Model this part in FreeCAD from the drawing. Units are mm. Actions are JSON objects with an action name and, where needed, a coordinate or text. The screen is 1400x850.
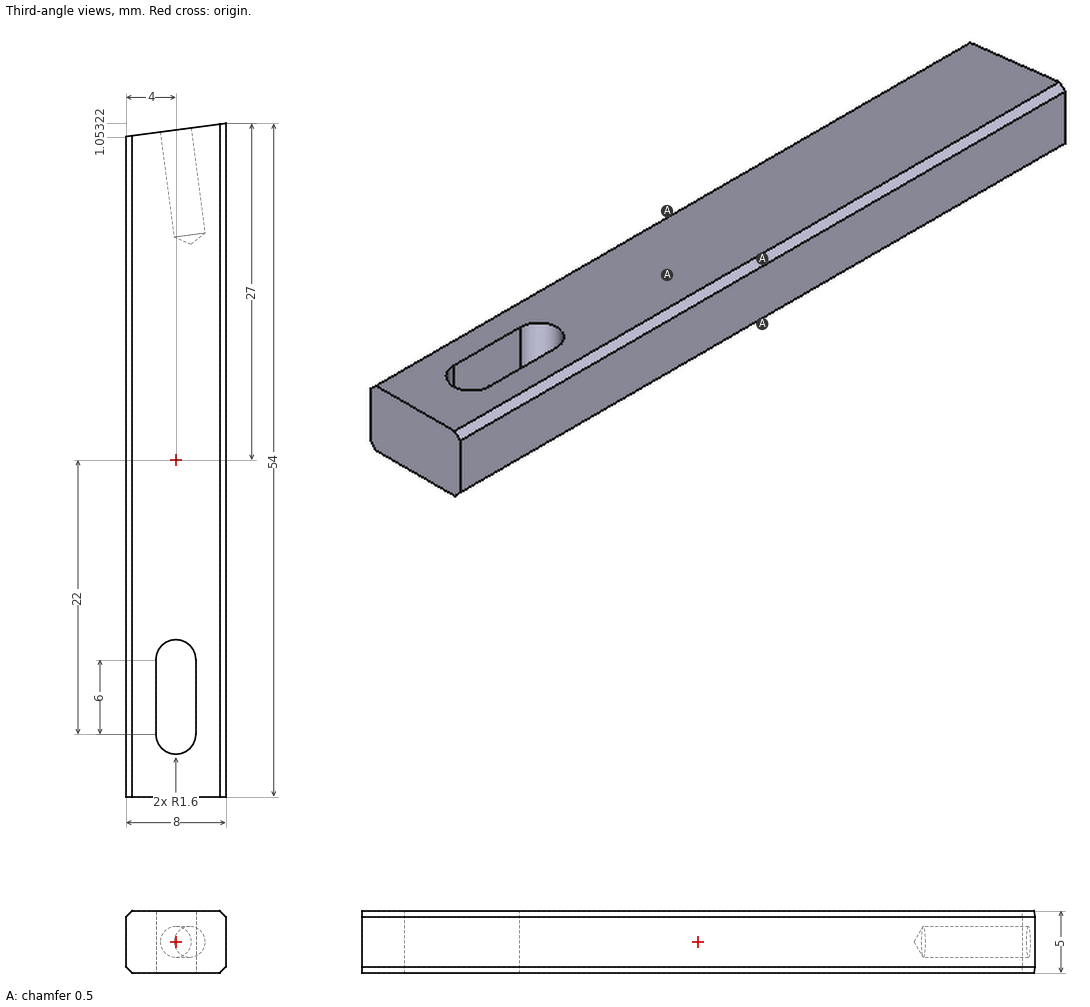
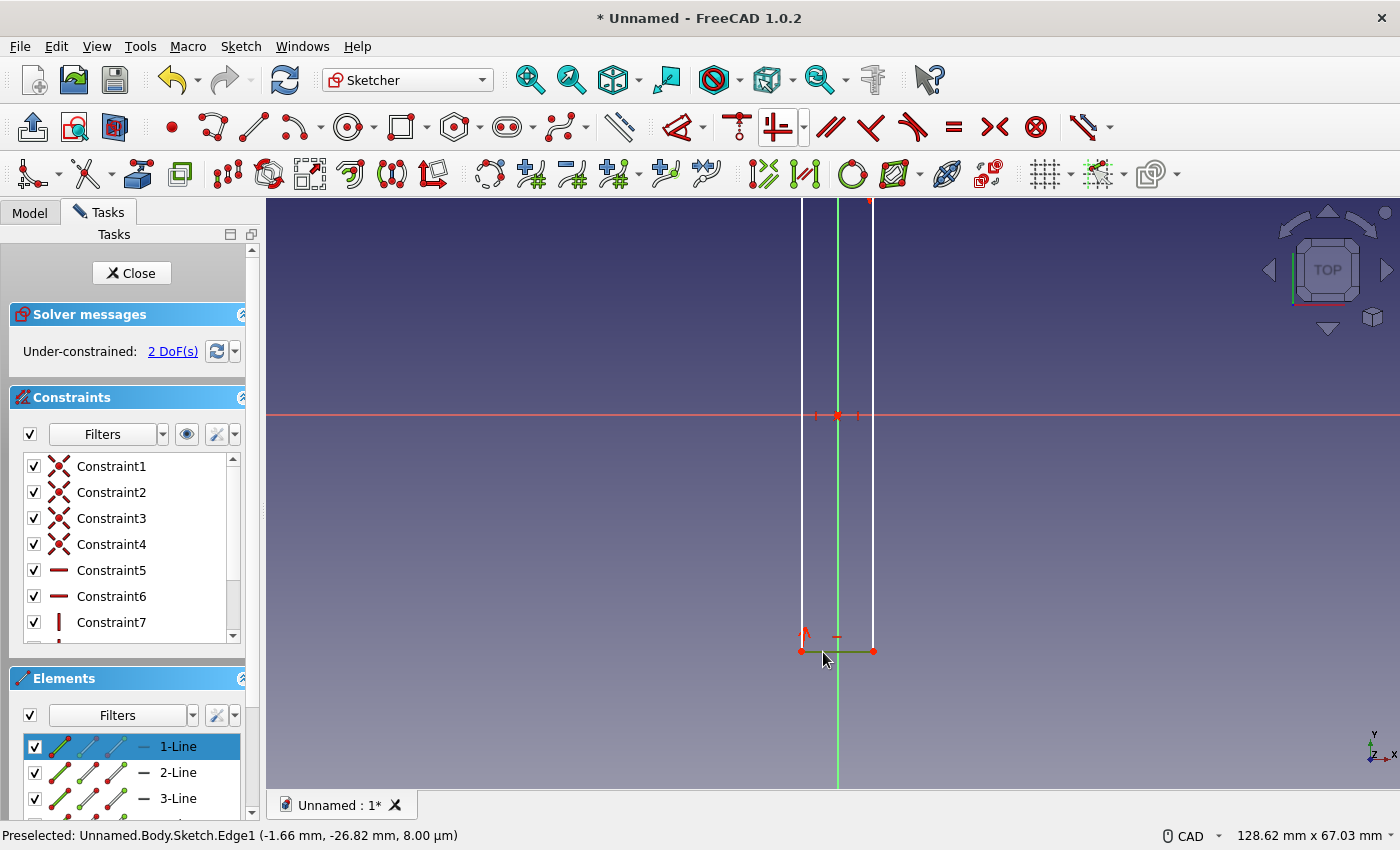
{"action": "key", "text": "l"}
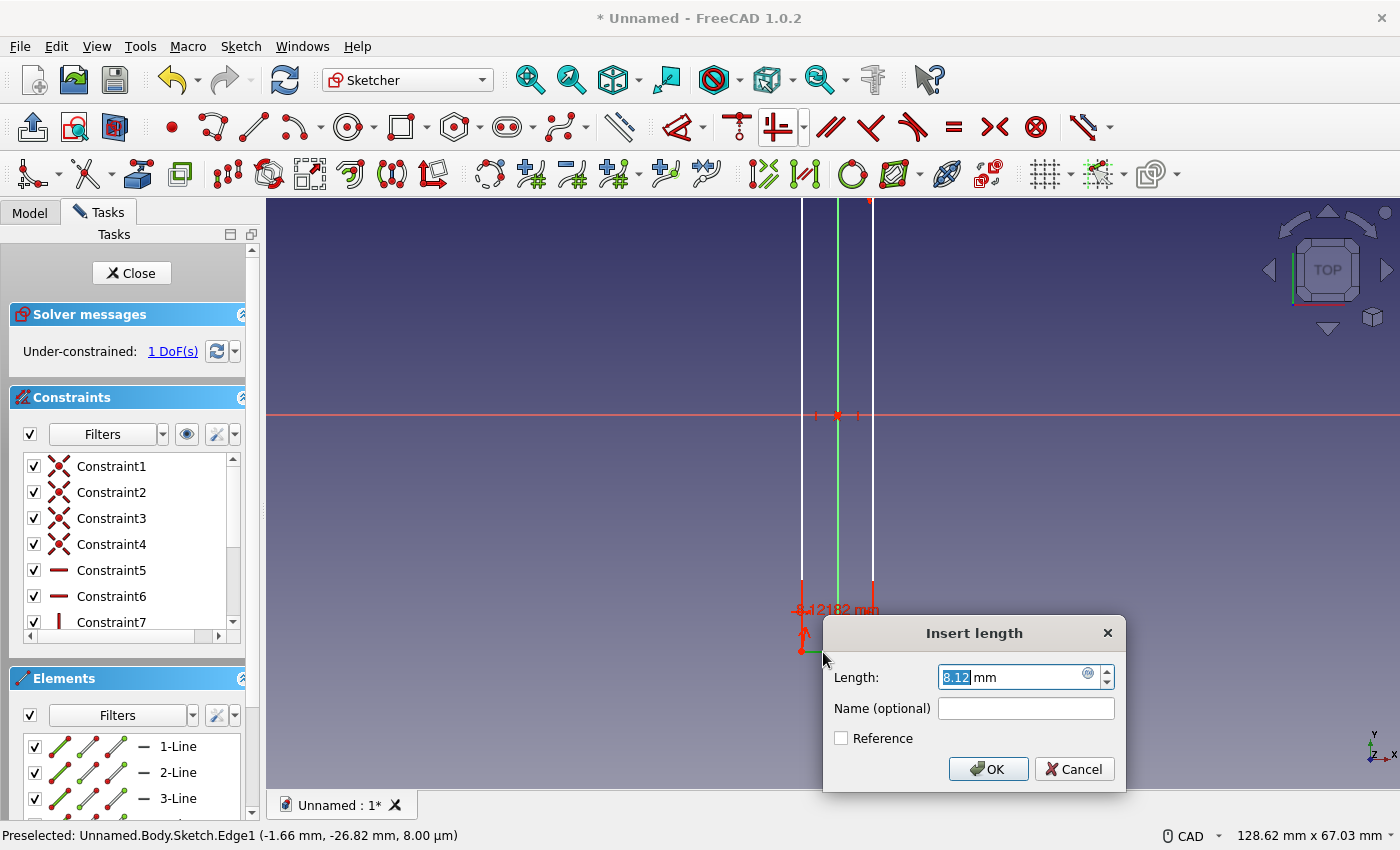
{"action": "type", "text": "8"}
{"action": "key", "text": "Return"}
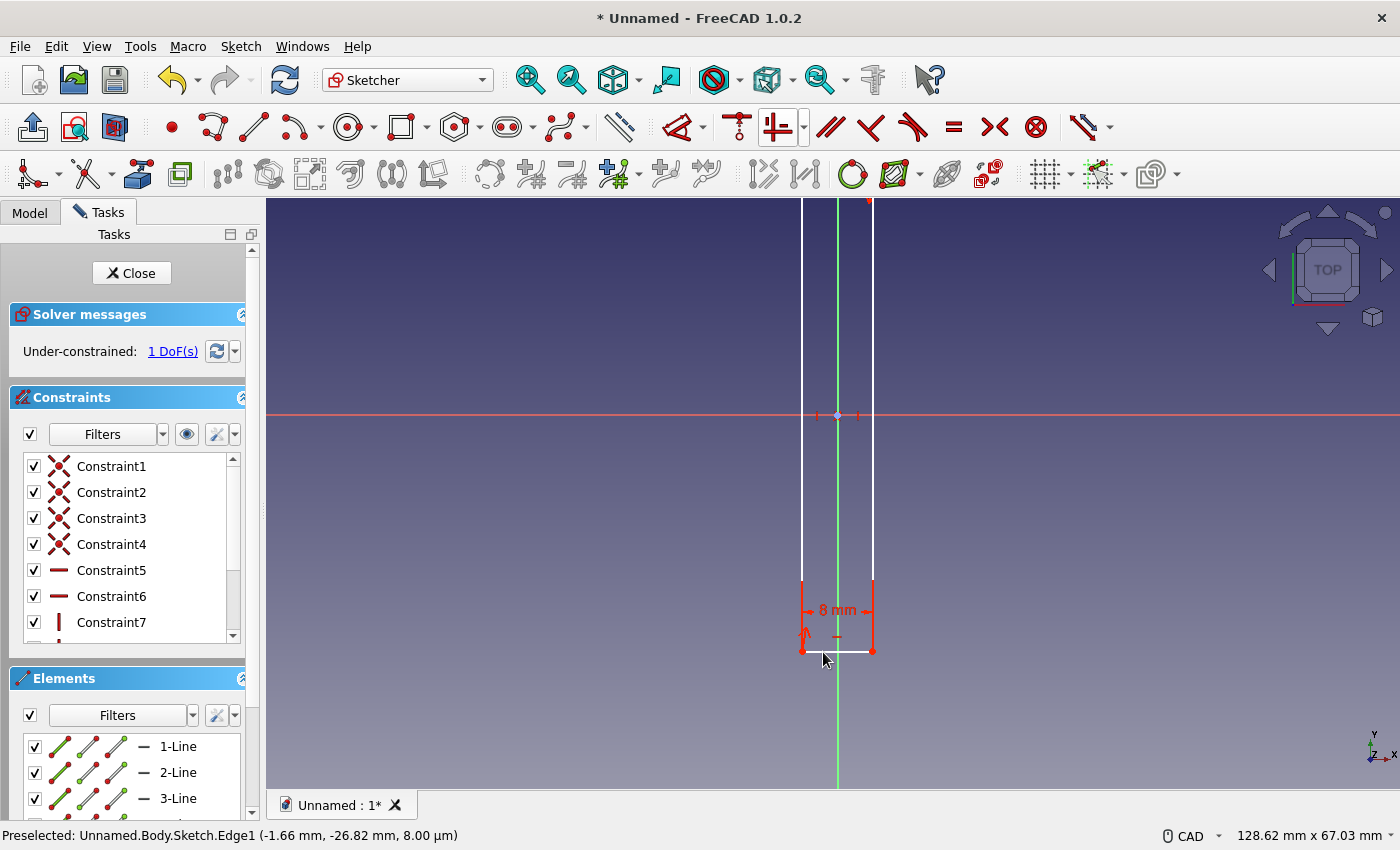
{"action": "left_click", "coordinate": [873, 510]}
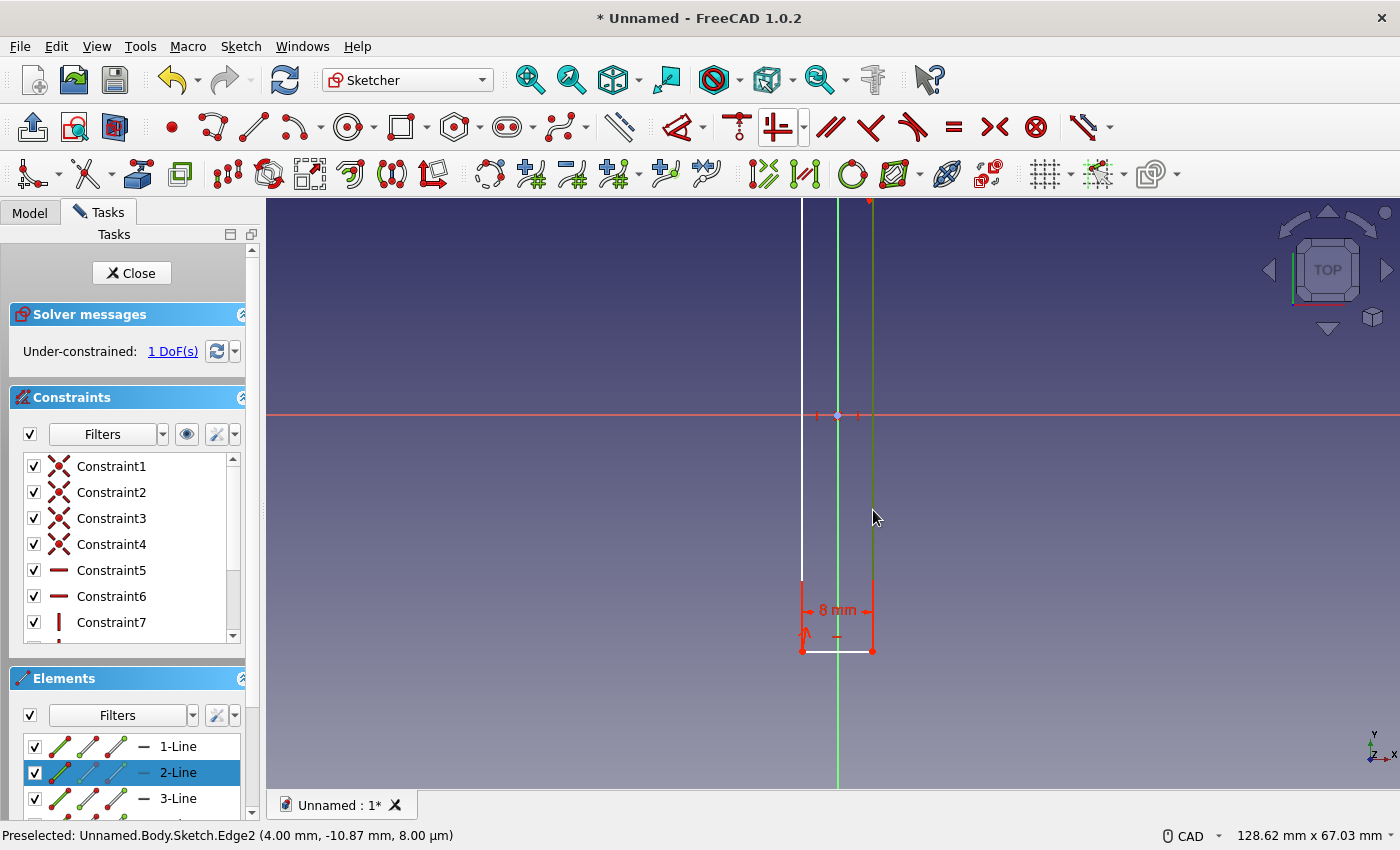
{"action": "key", "text": "i"}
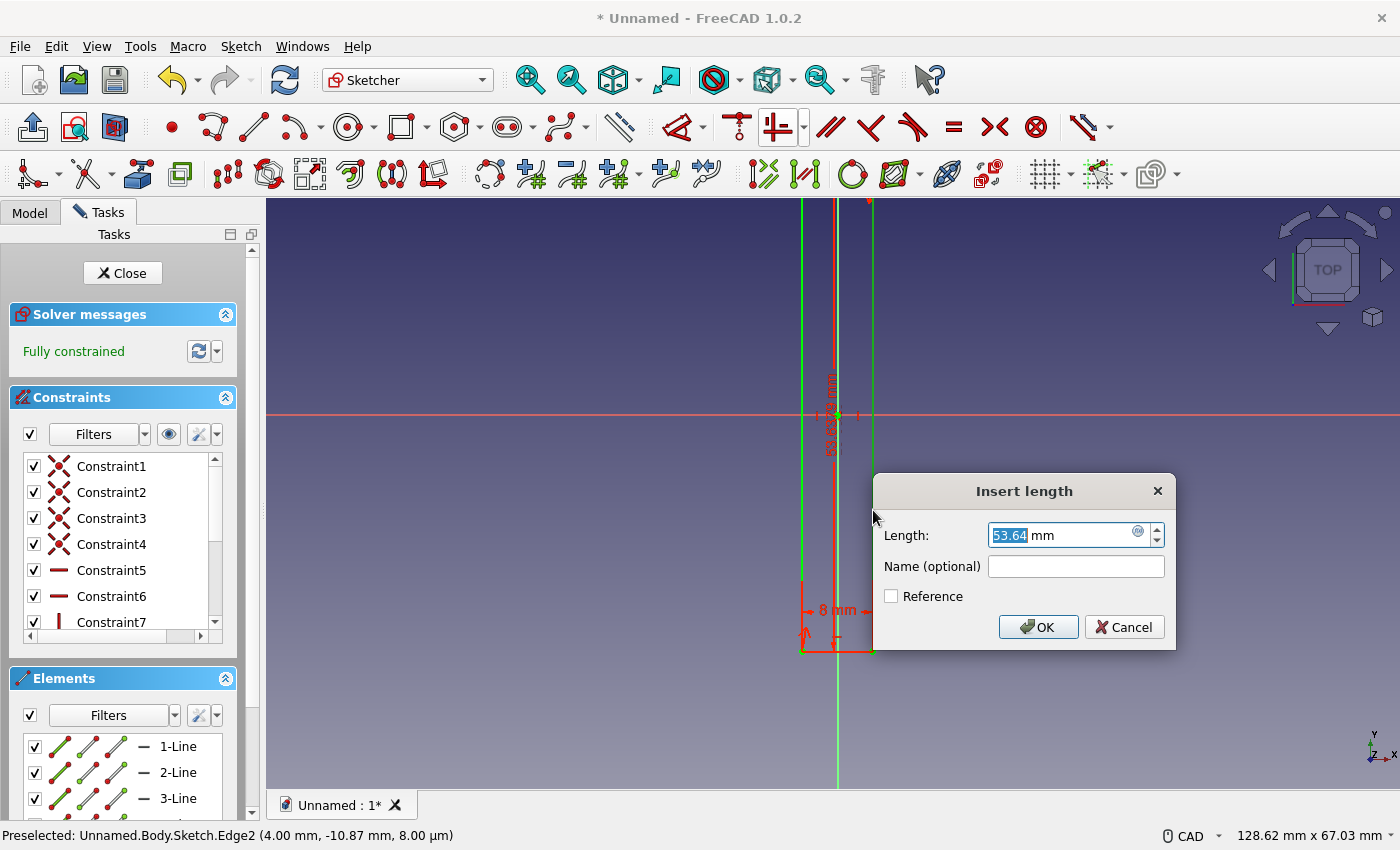
{"action": "type", "text": "54"}
{"action": "key", "text": "Return"}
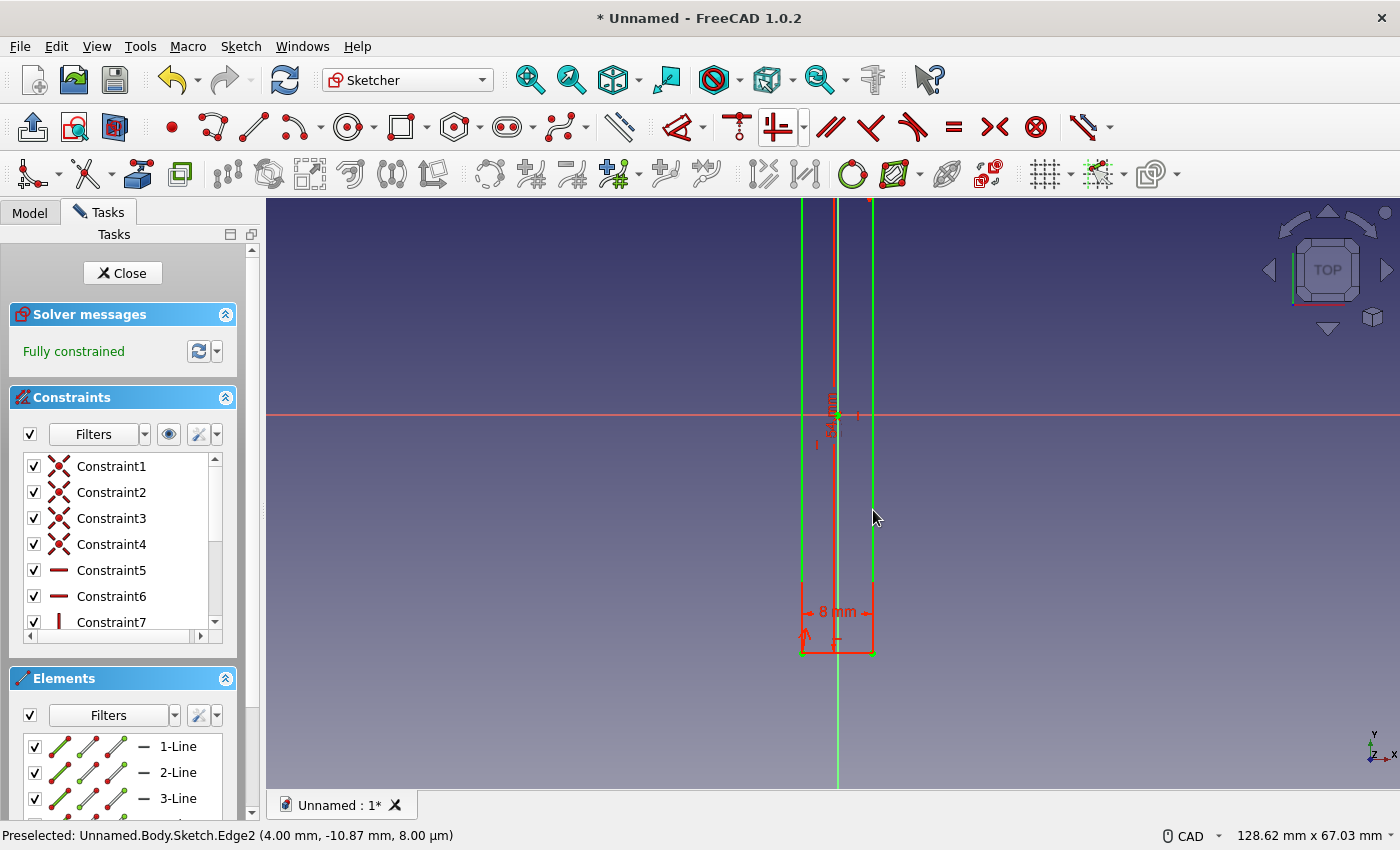
{"action": "left_click", "coordinate": [123, 273]}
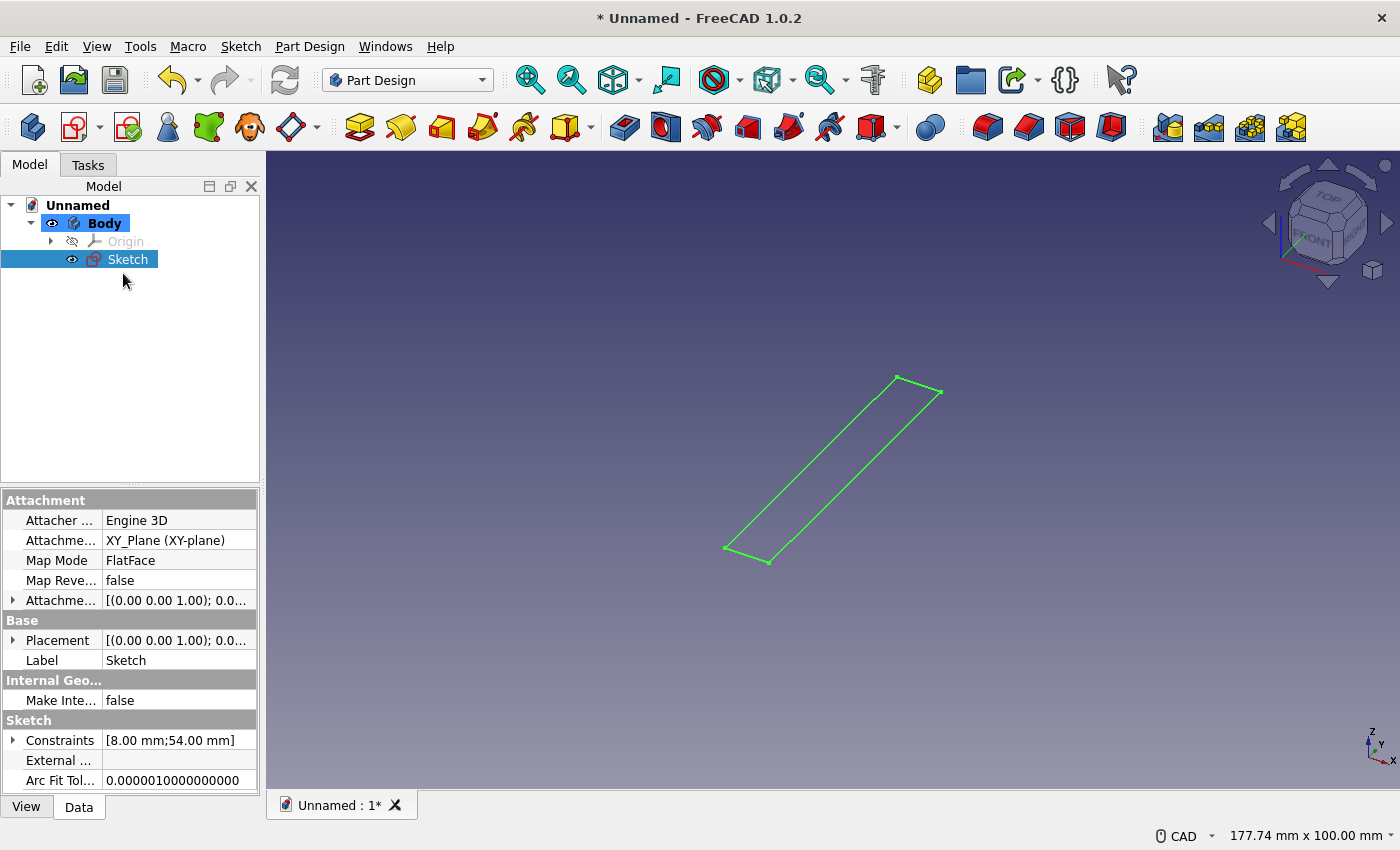
{"action": "left_click", "coordinate": [360, 128]}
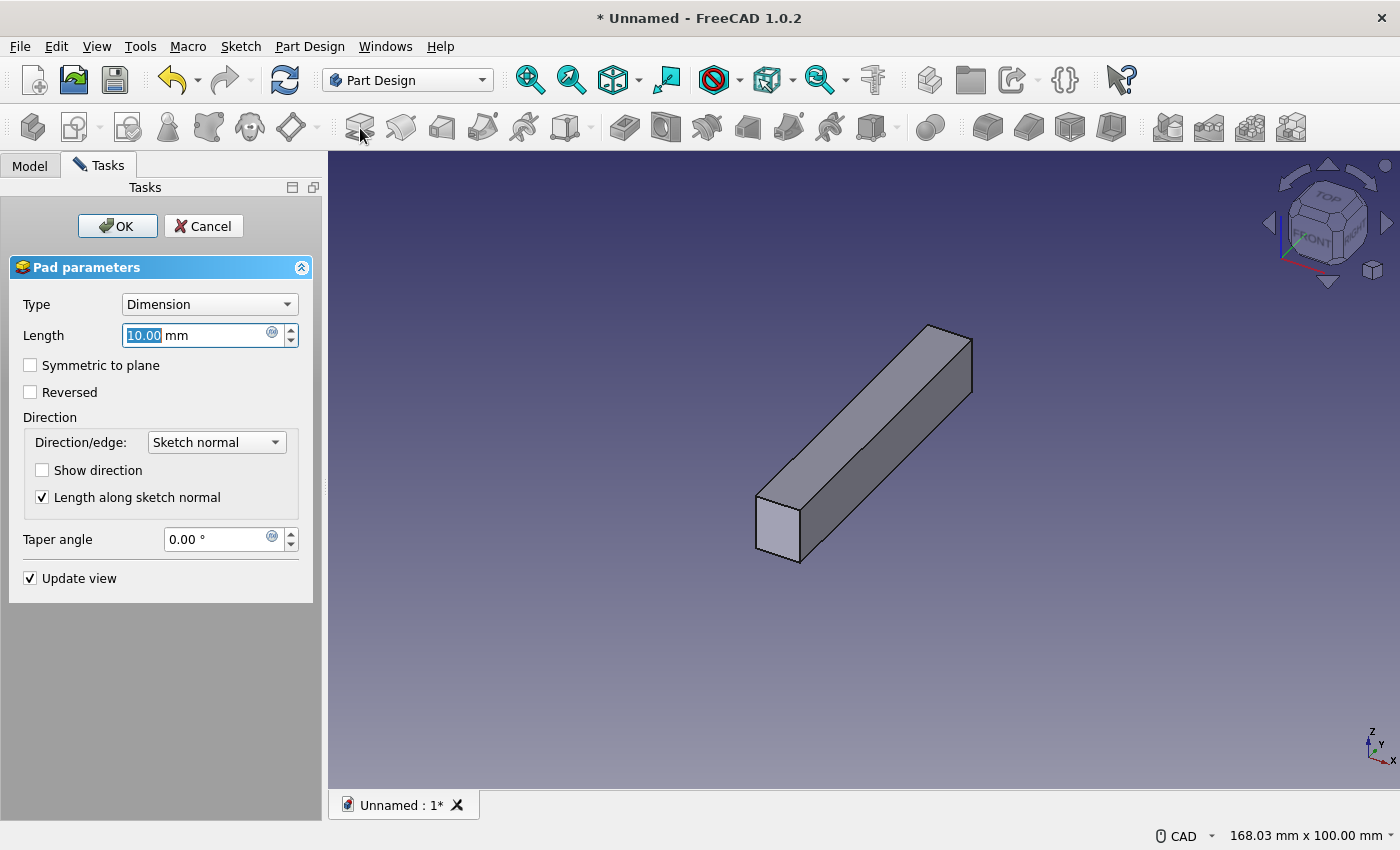
{"action": "type", "text": "5"}
{"action": "key", "text": "Tab"}